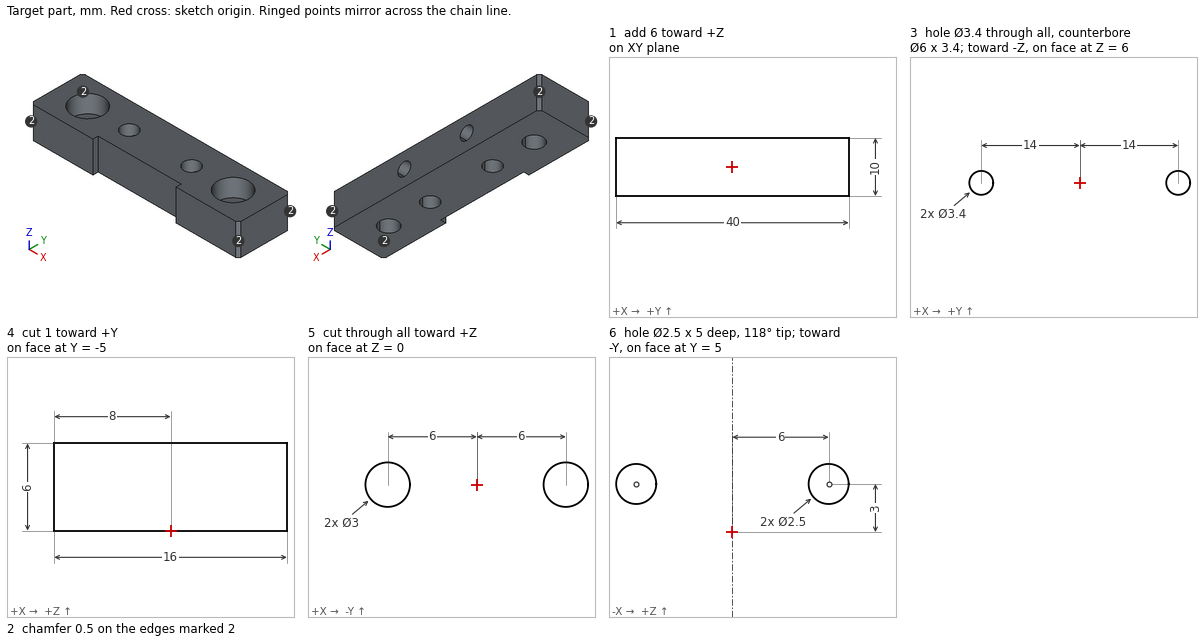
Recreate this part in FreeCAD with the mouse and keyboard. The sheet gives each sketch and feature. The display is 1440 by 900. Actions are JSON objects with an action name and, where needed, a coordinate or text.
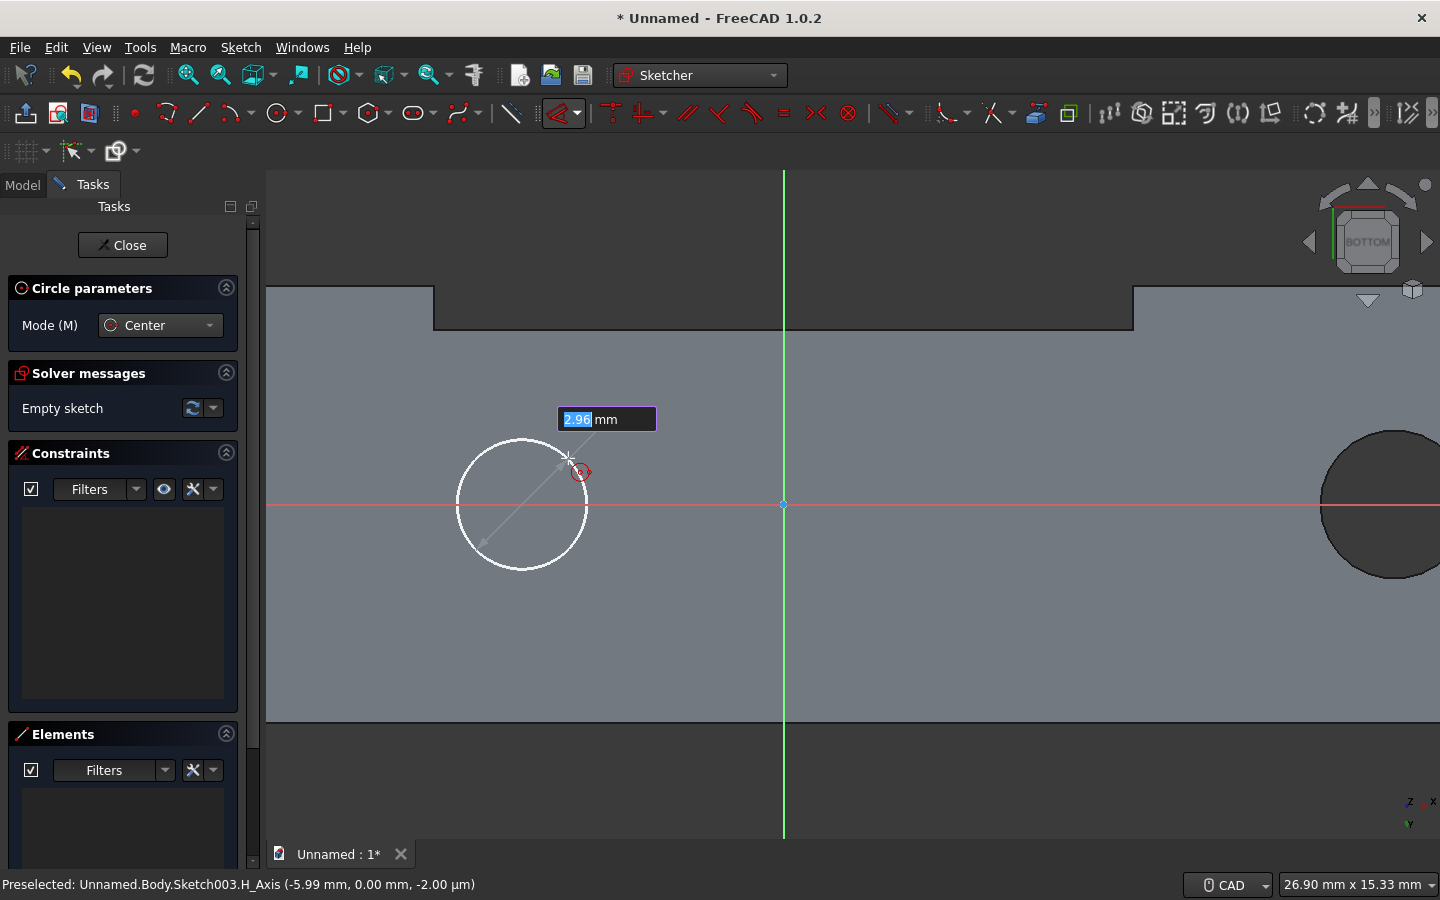
{"action": "type", "text": "3"}
{"action": "key", "text": "Return"}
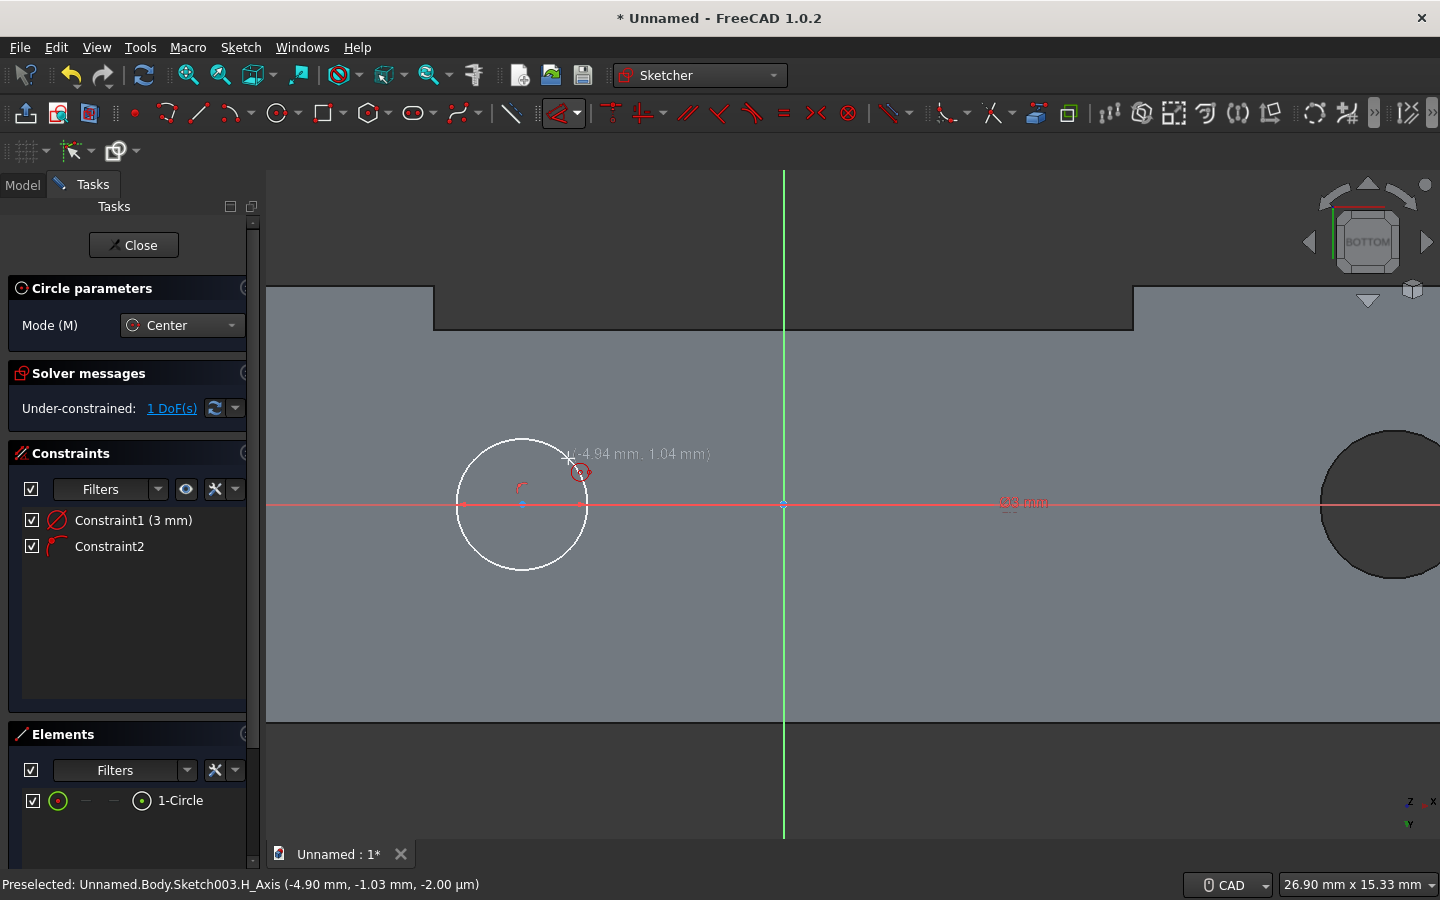
{"action": "left_click", "coordinate": [1045, 504]}
{"action": "mouse_move", "coordinate": [1092, 458]}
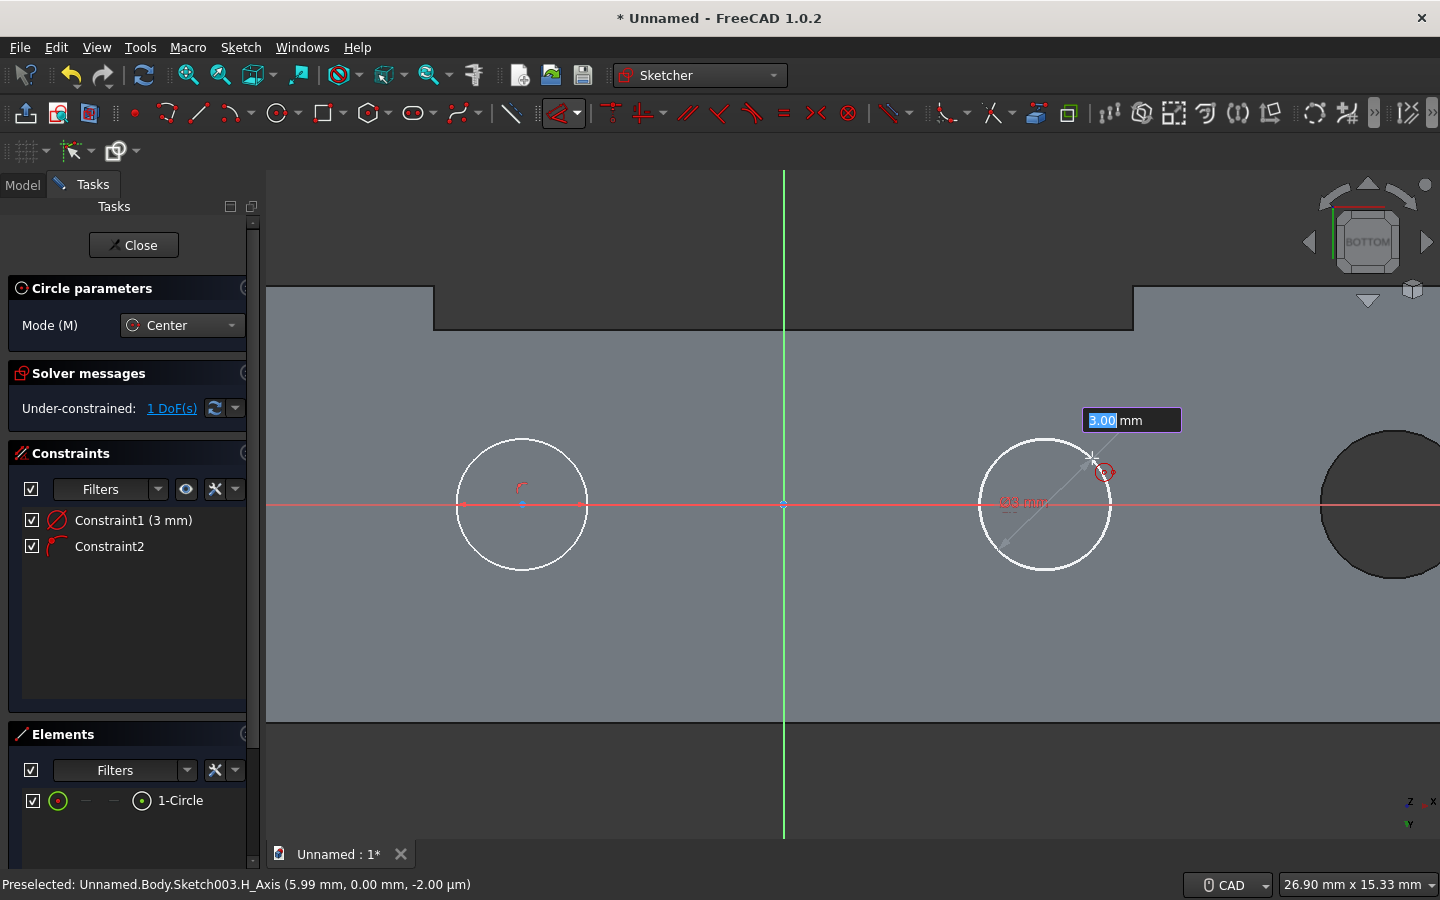
{"action": "type", "text": "3"}
{"action": "key", "text": "Return"}
{"action": "key", "text": "Escape"}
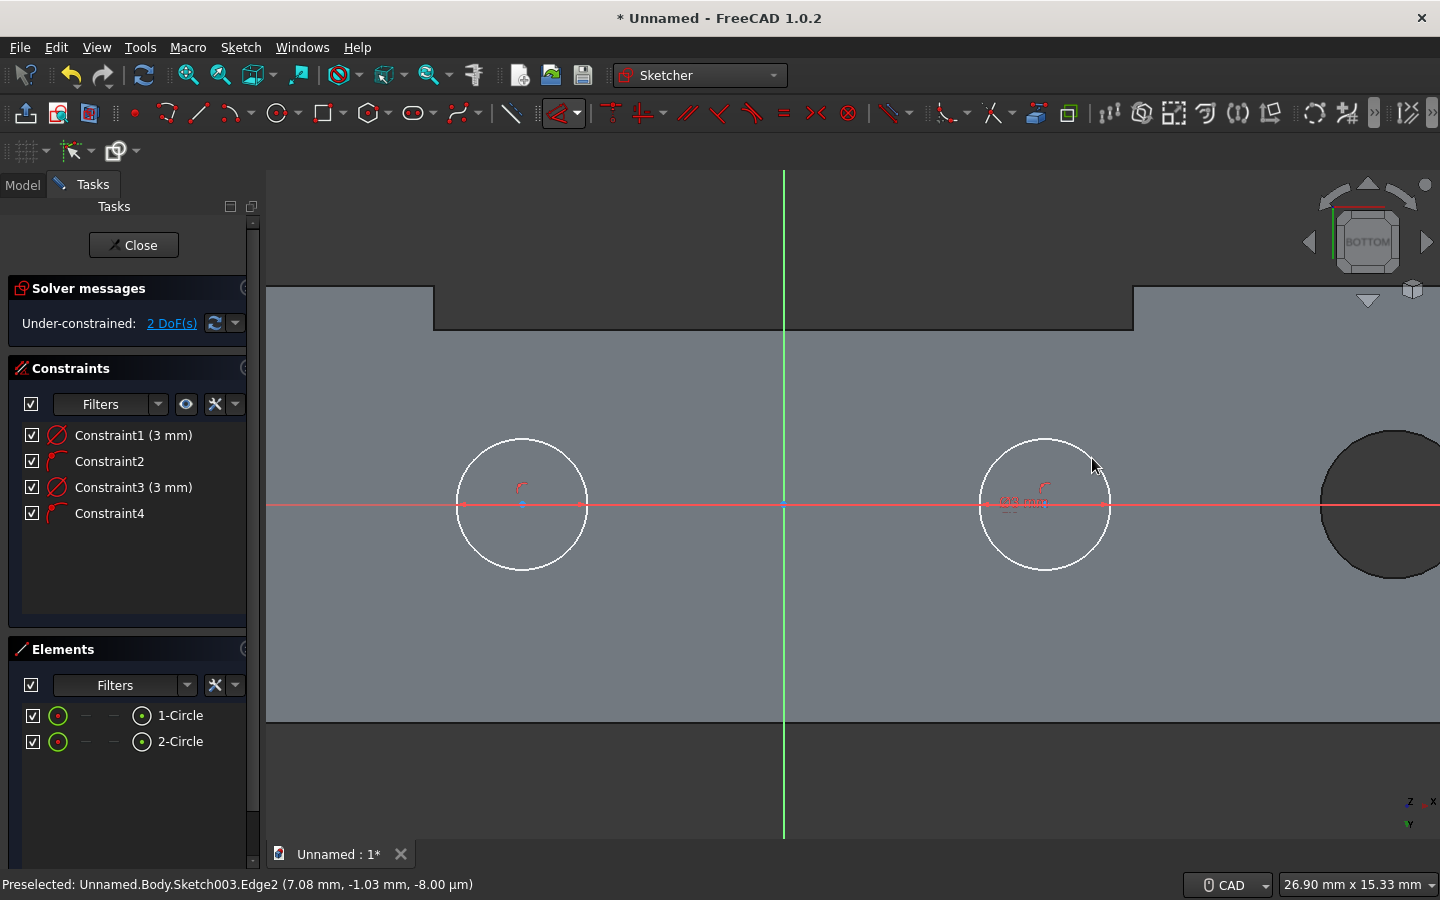
{"action": "left_click", "coordinate": [522, 504]}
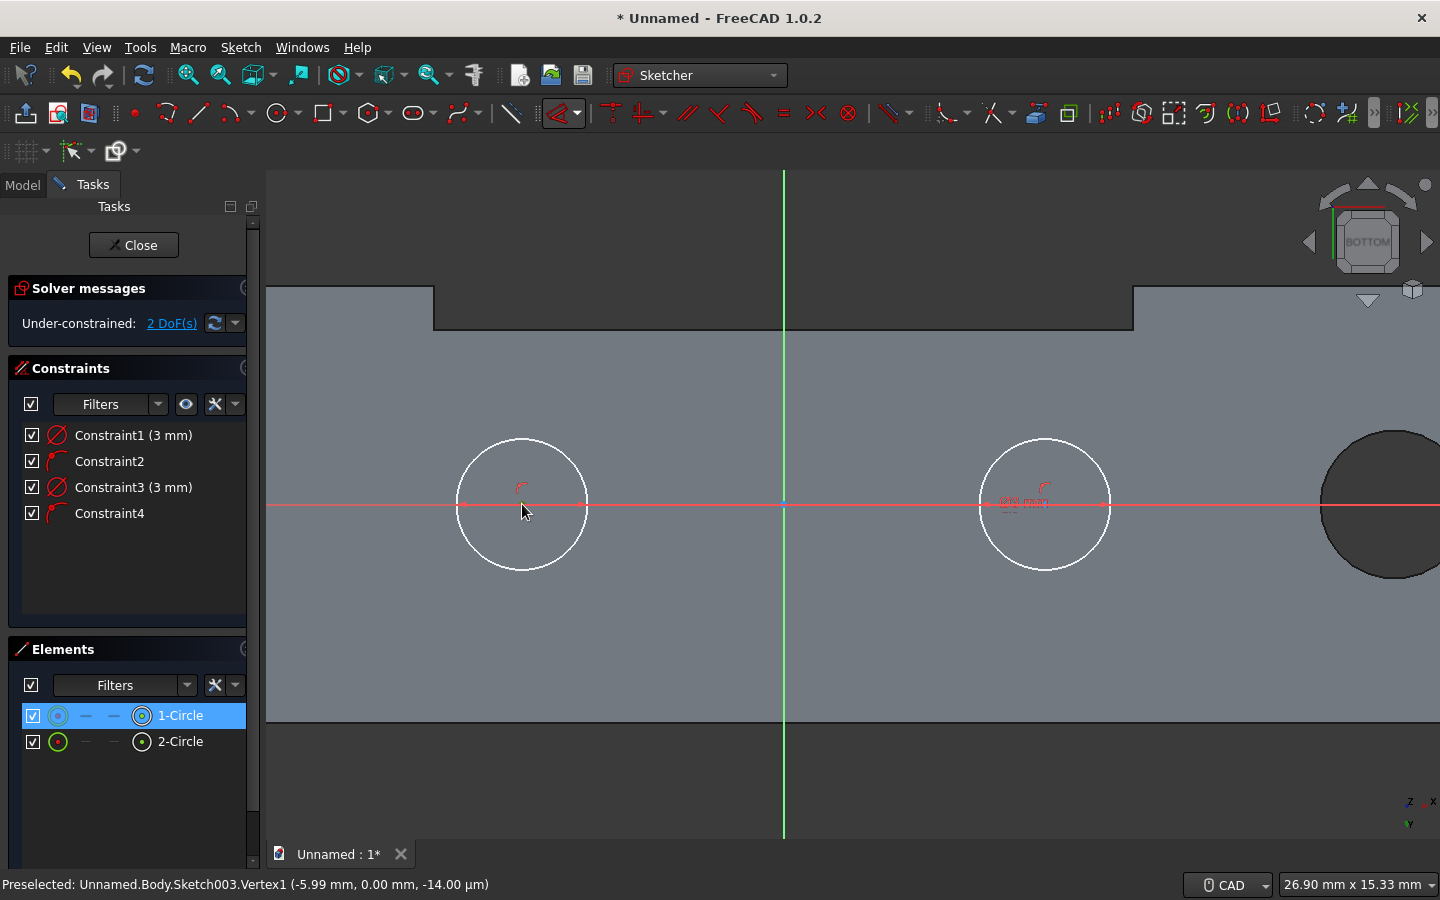
{"action": "key", "text": "l"}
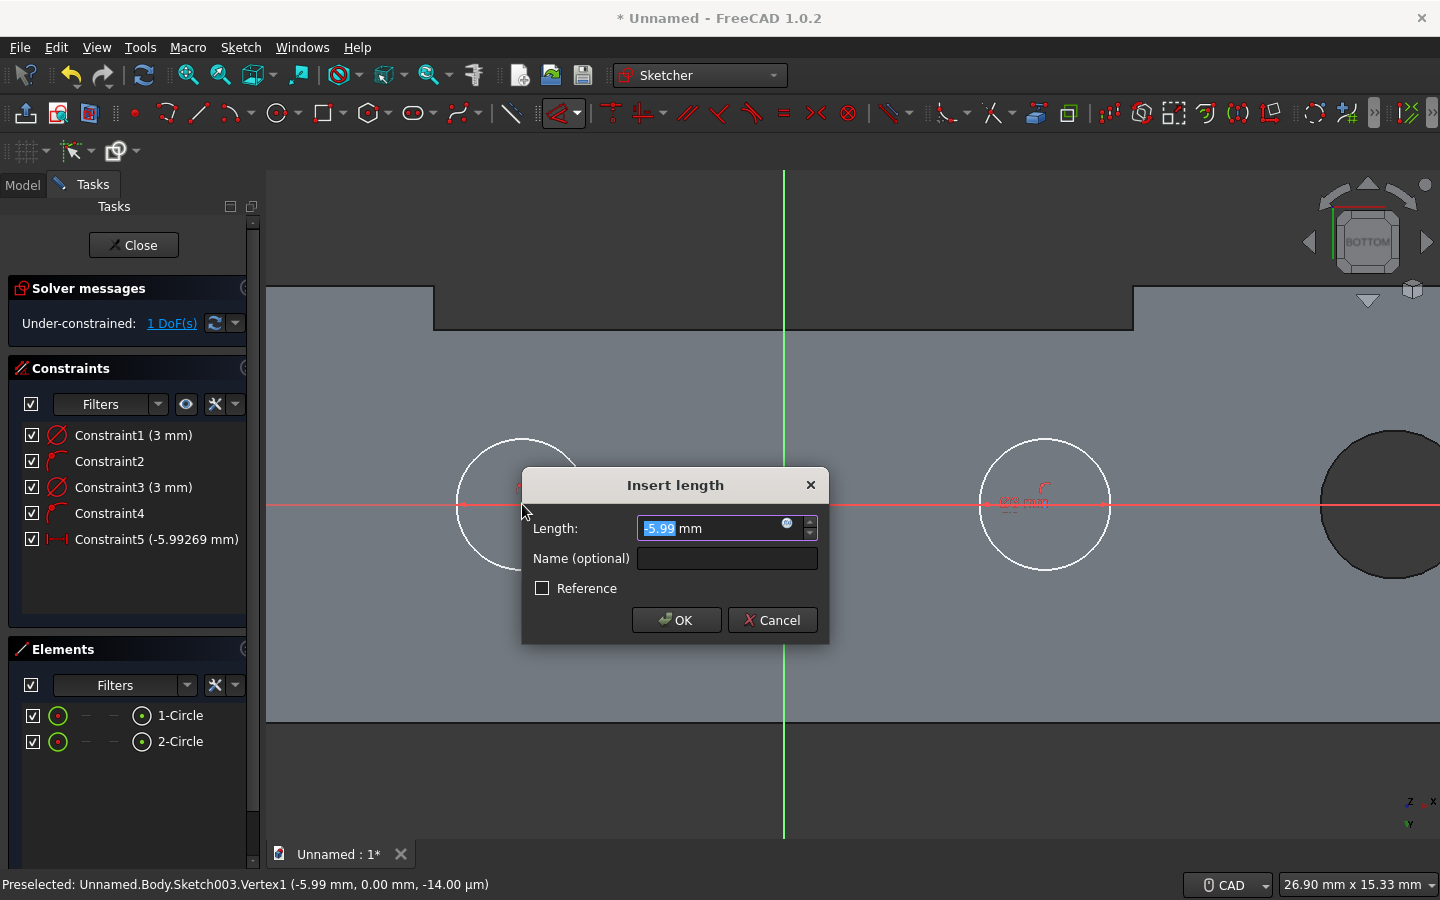
{"action": "type", "text": "-6"}
{"action": "key", "text": "Return"}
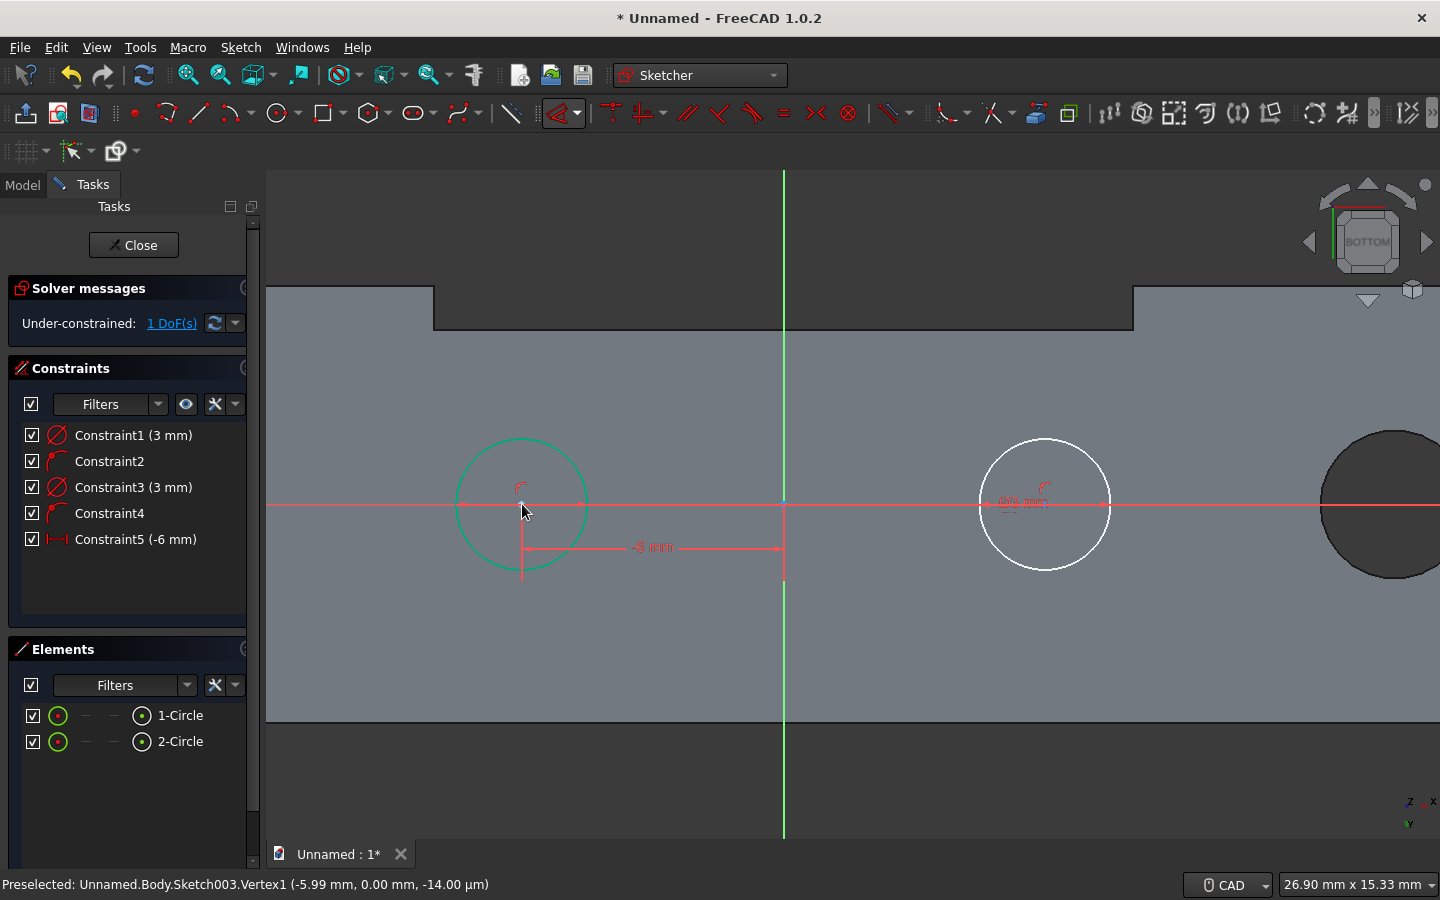
{"action": "left_click", "coordinate": [1045, 504]}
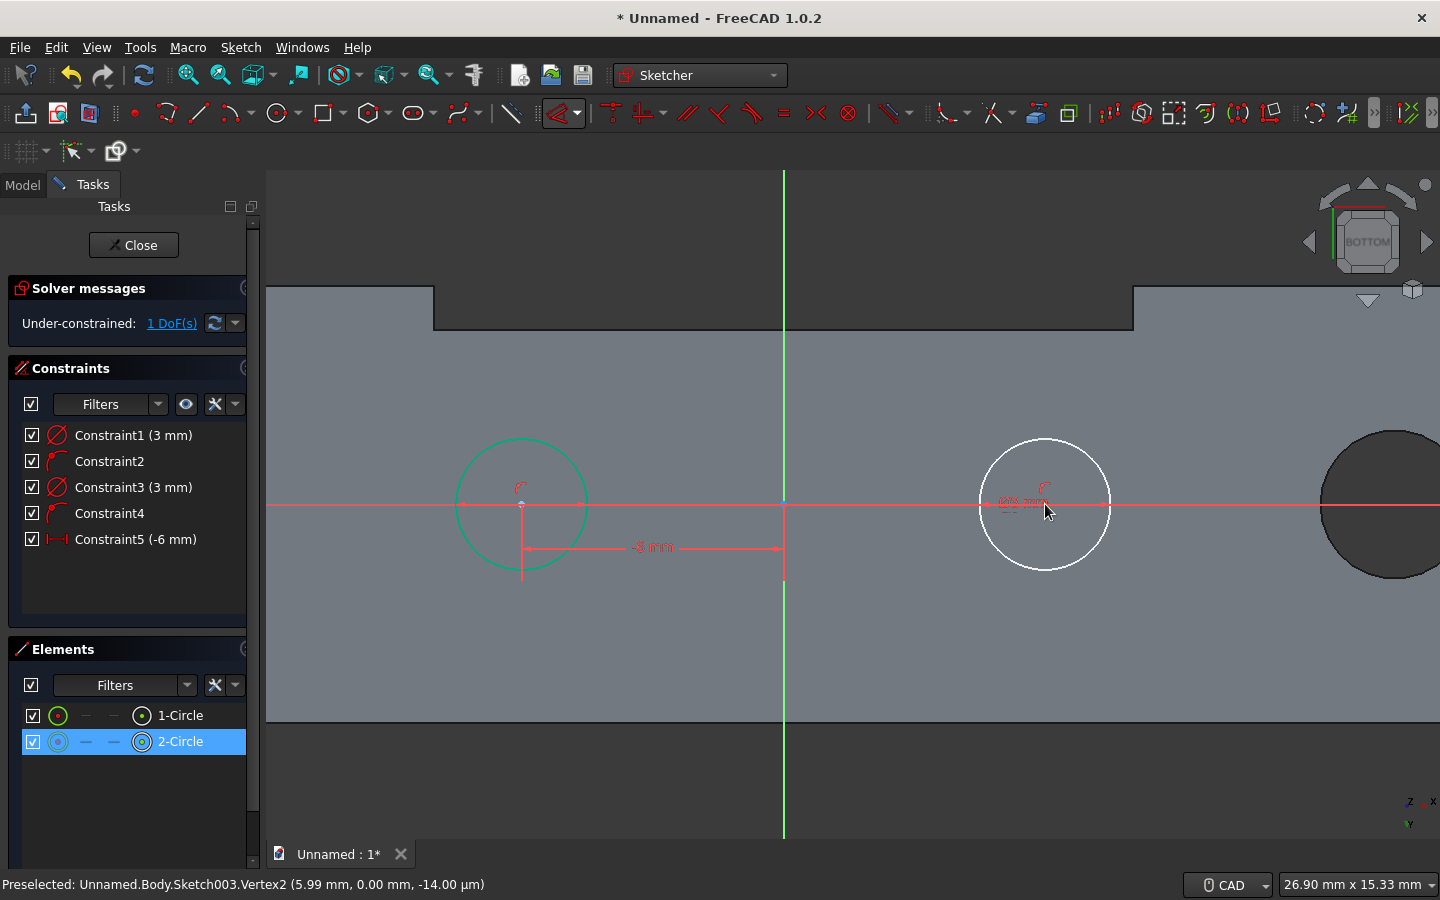
{"action": "left_click", "coordinate": [580, 114]}